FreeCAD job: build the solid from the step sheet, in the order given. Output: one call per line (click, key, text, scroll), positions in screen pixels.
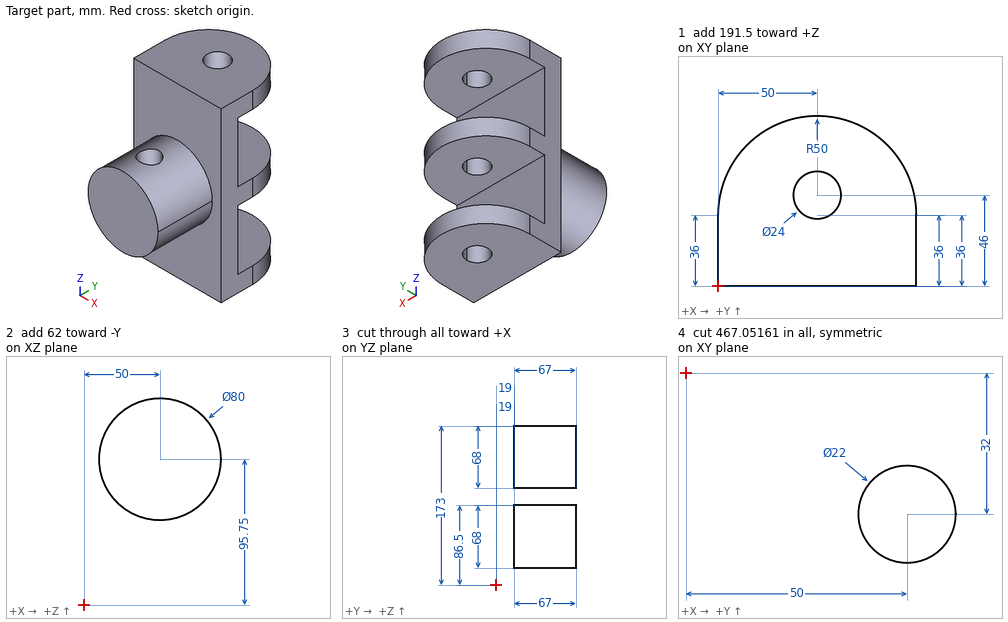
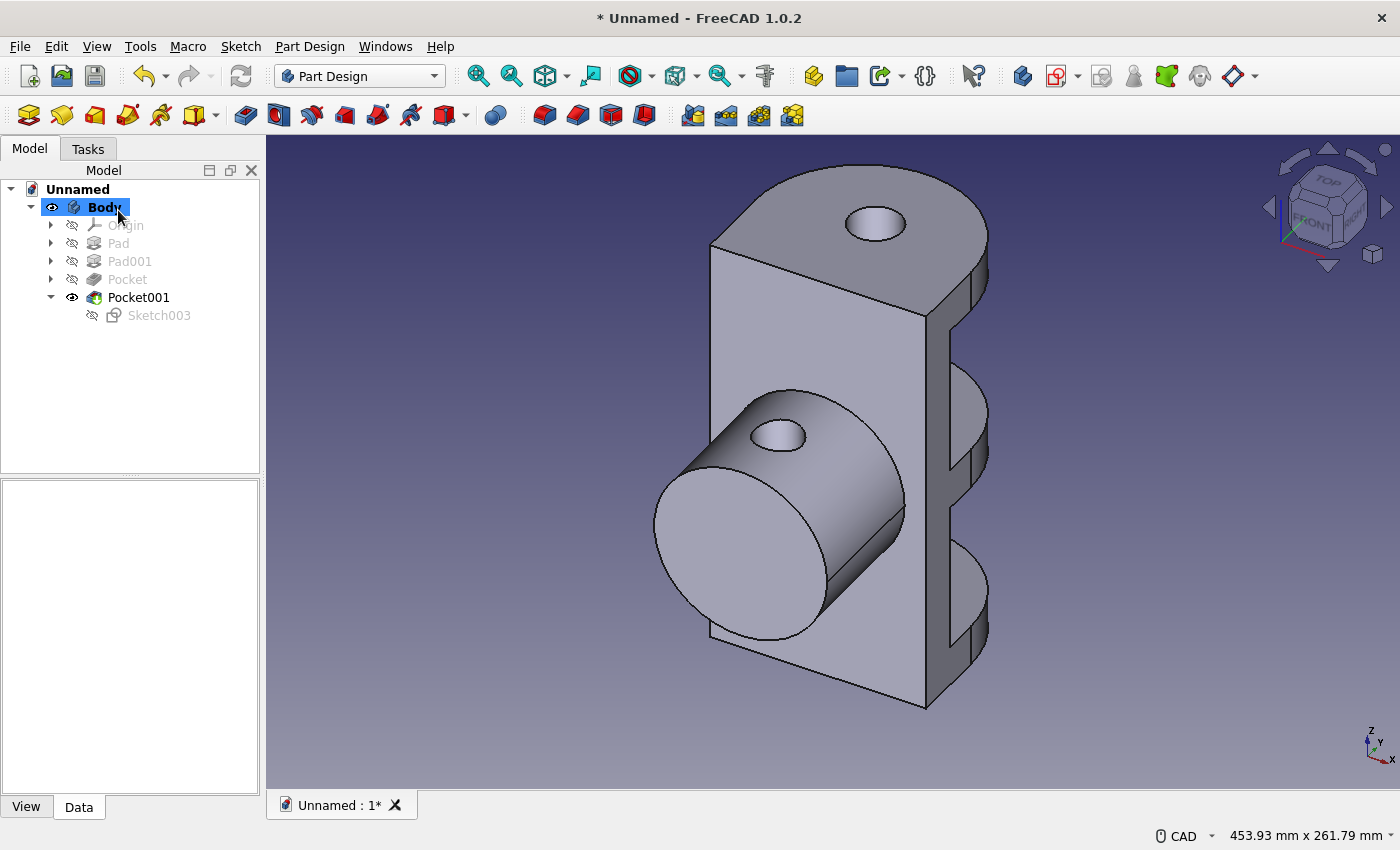
key(0)